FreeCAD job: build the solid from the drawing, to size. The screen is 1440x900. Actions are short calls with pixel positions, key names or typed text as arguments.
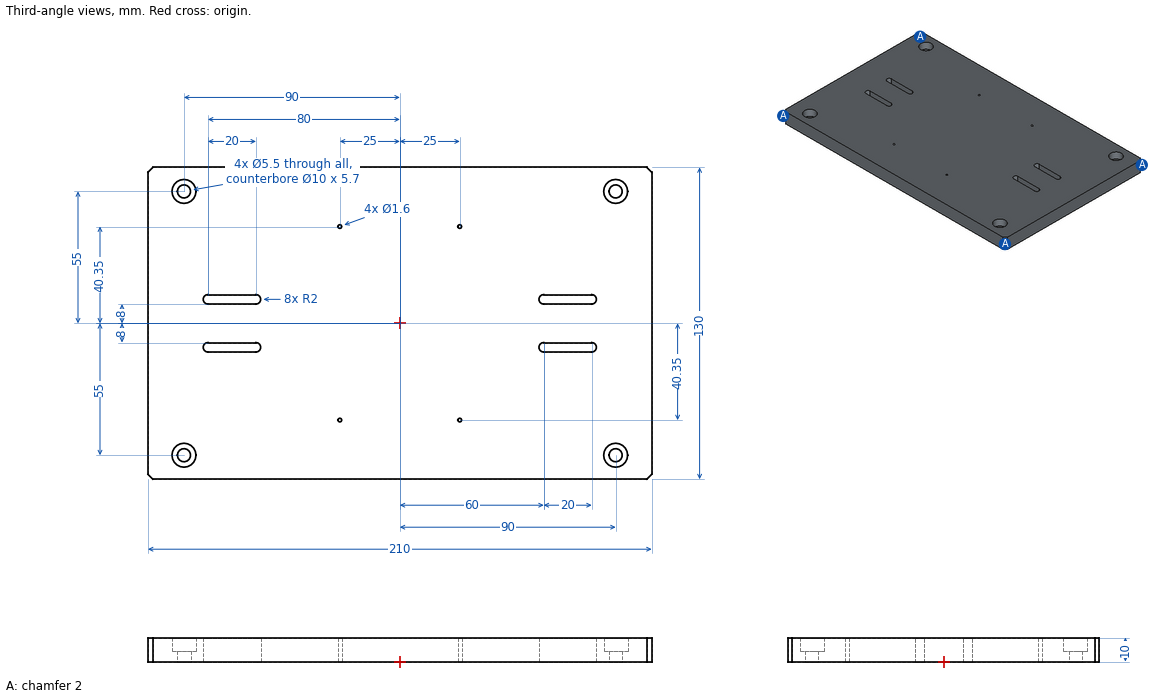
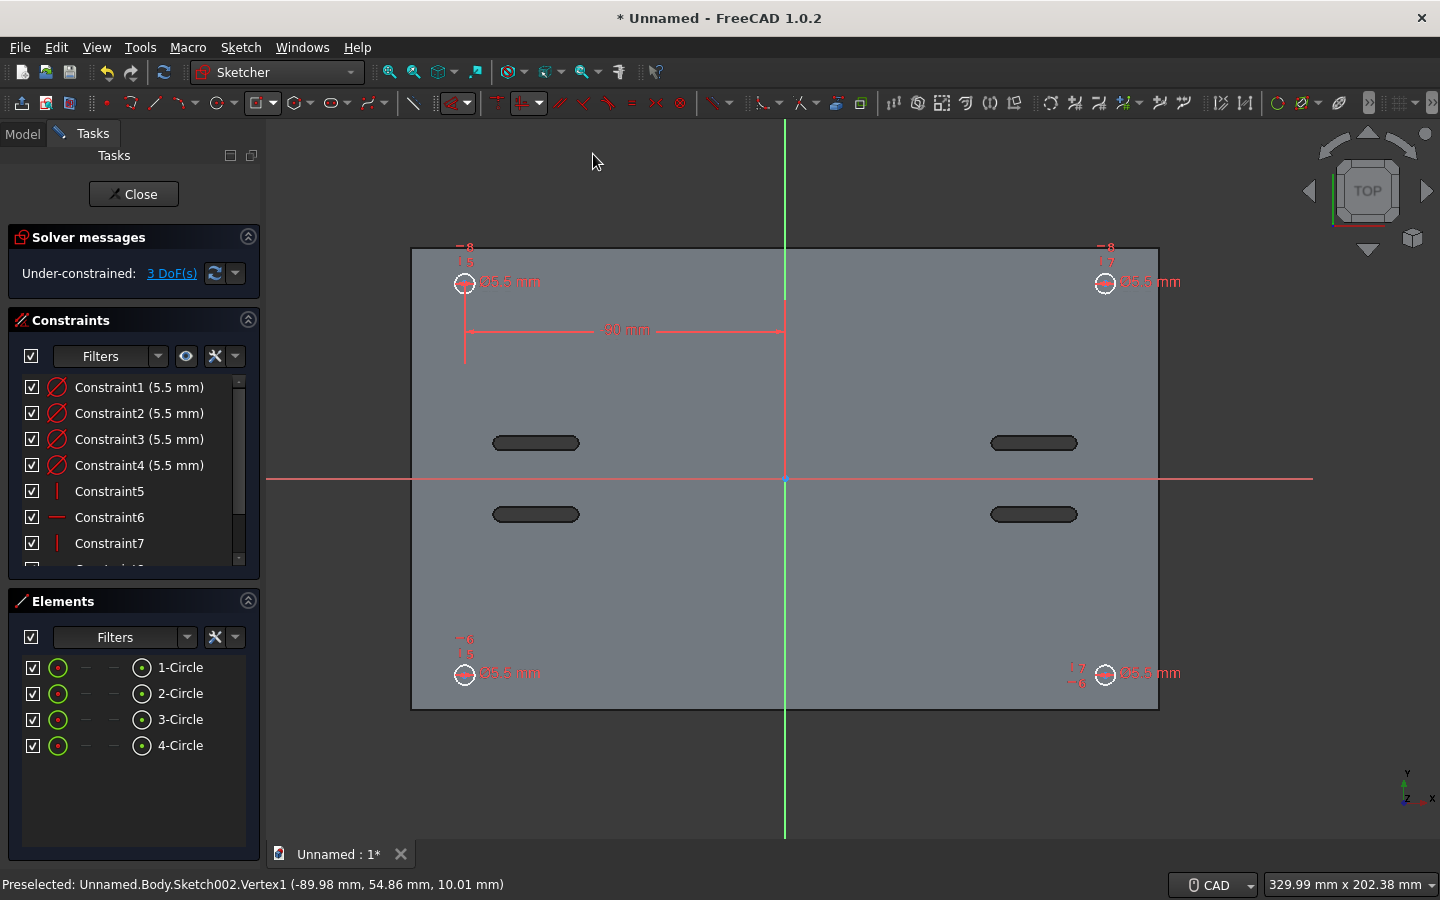
click(465, 284)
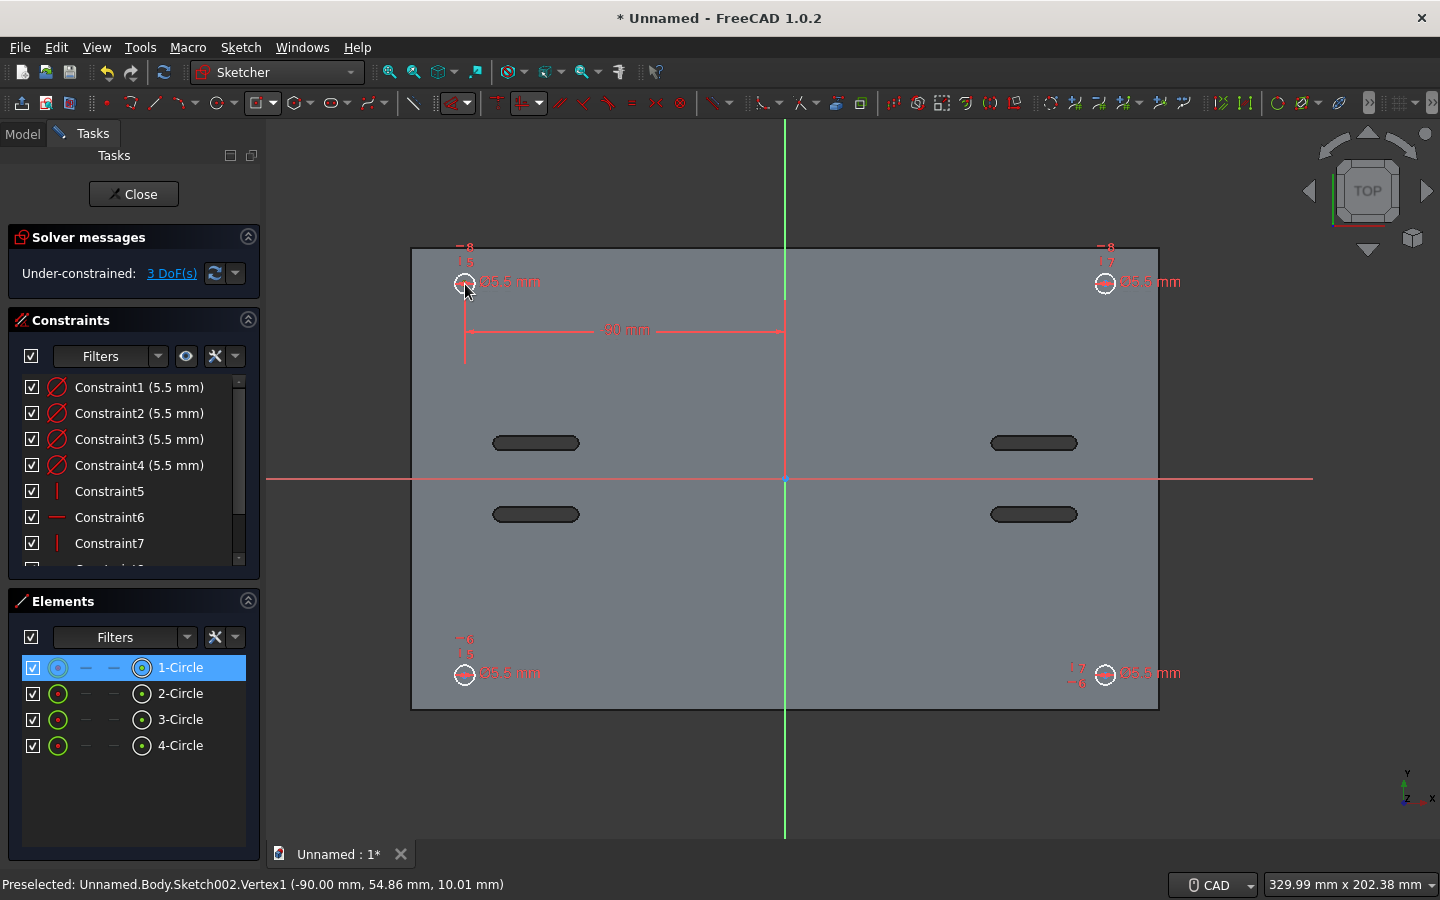
key(i)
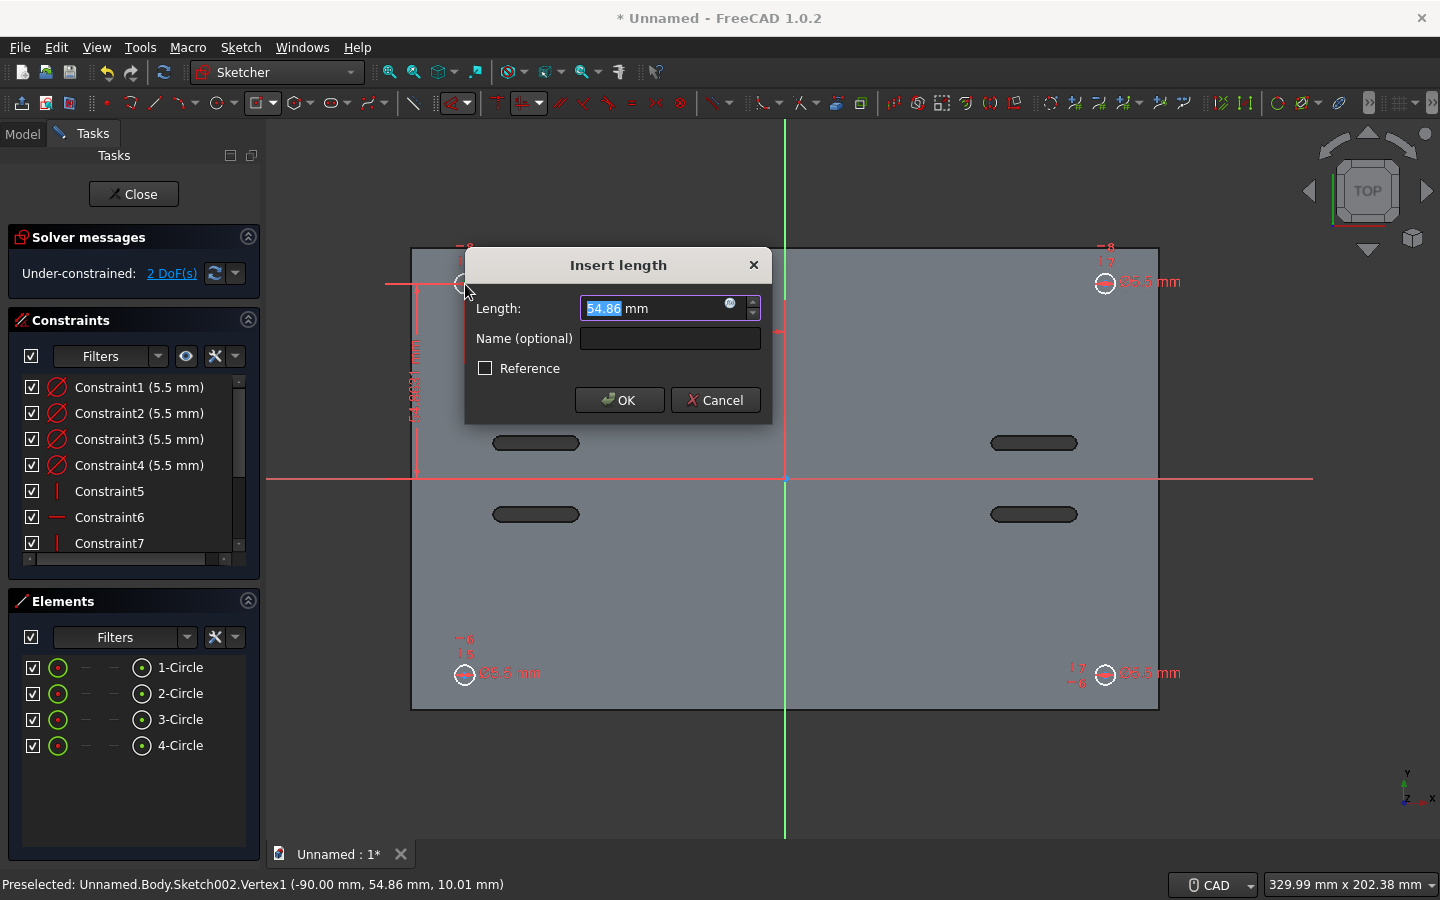
text(55)
key(Return)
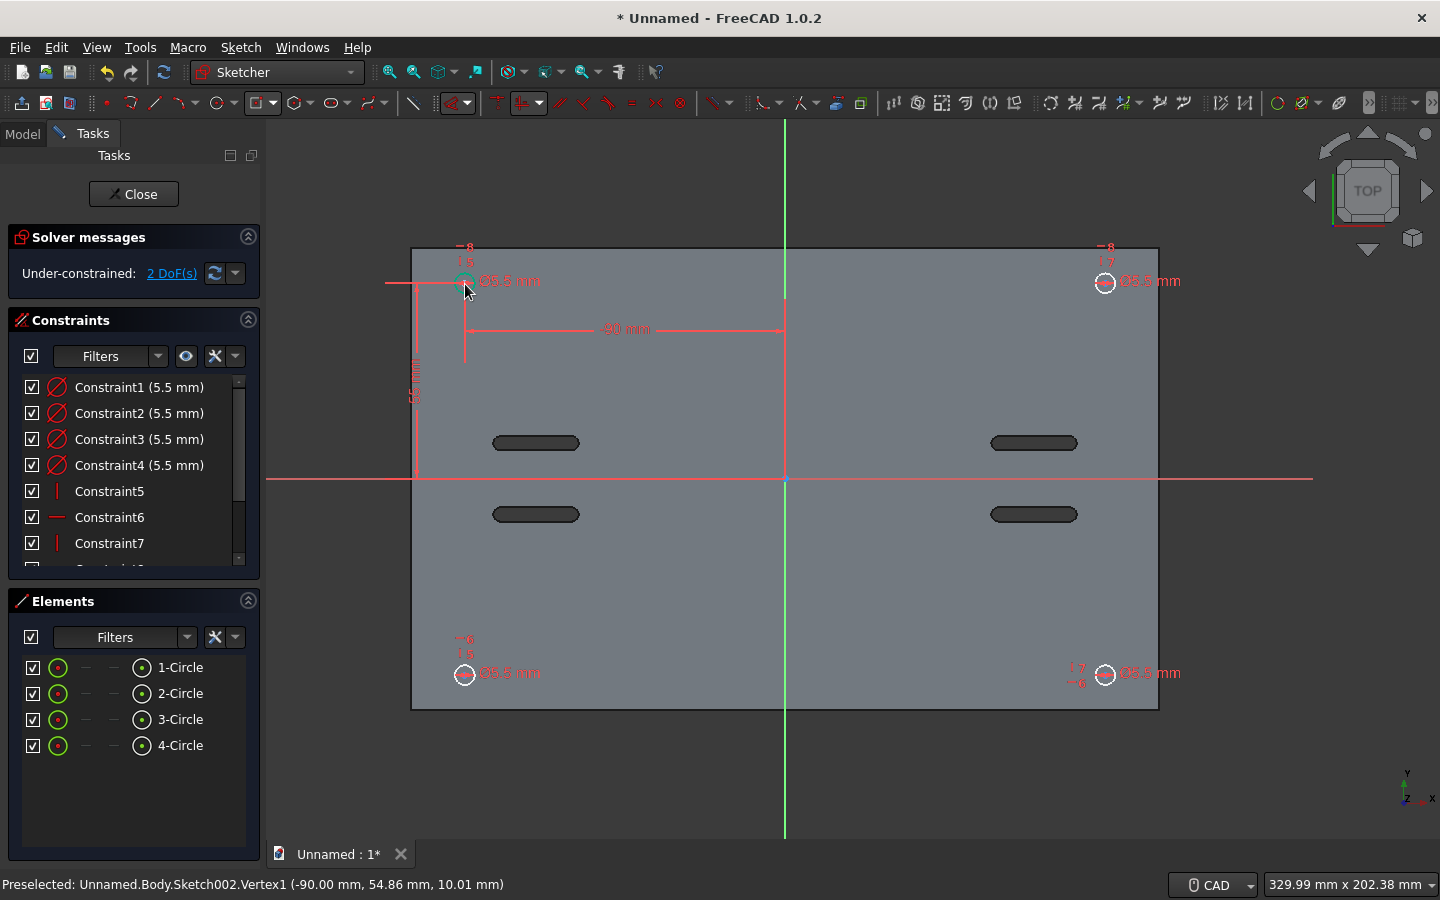
click(465, 675)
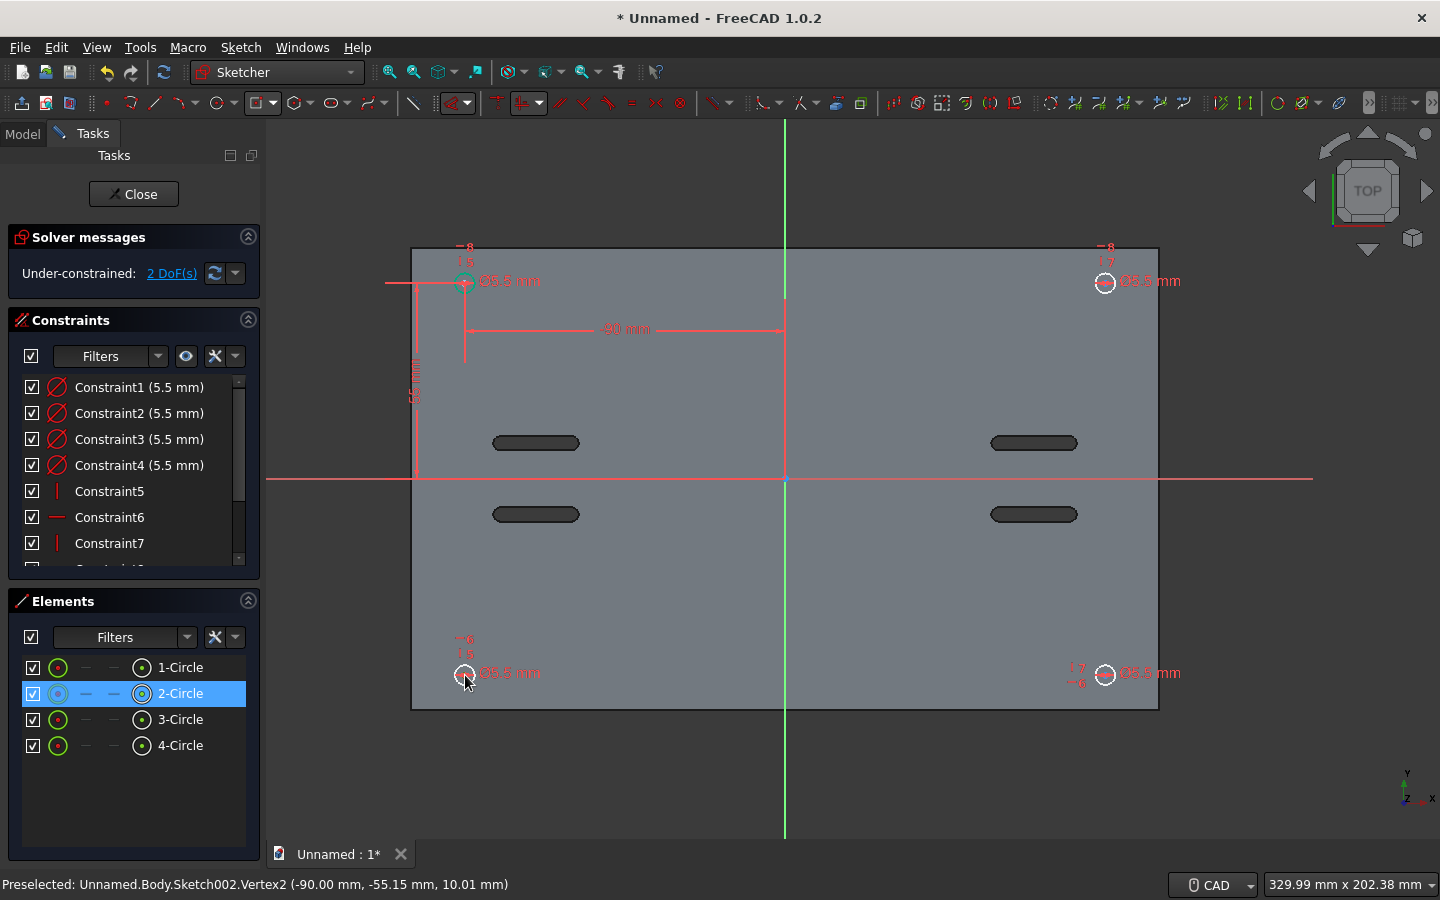
key(i)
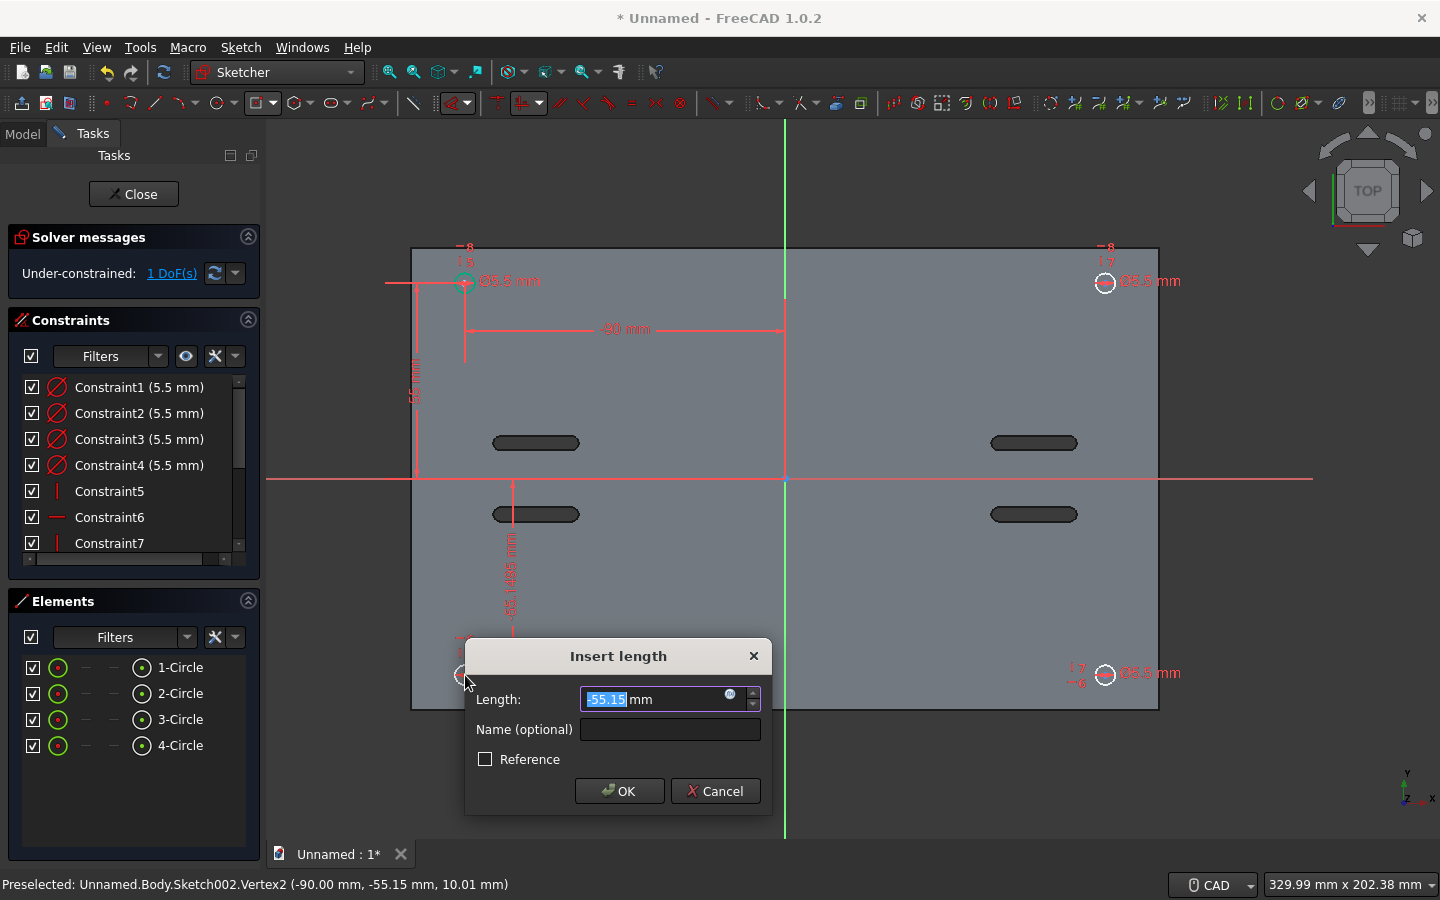
text(-55)
key(Return)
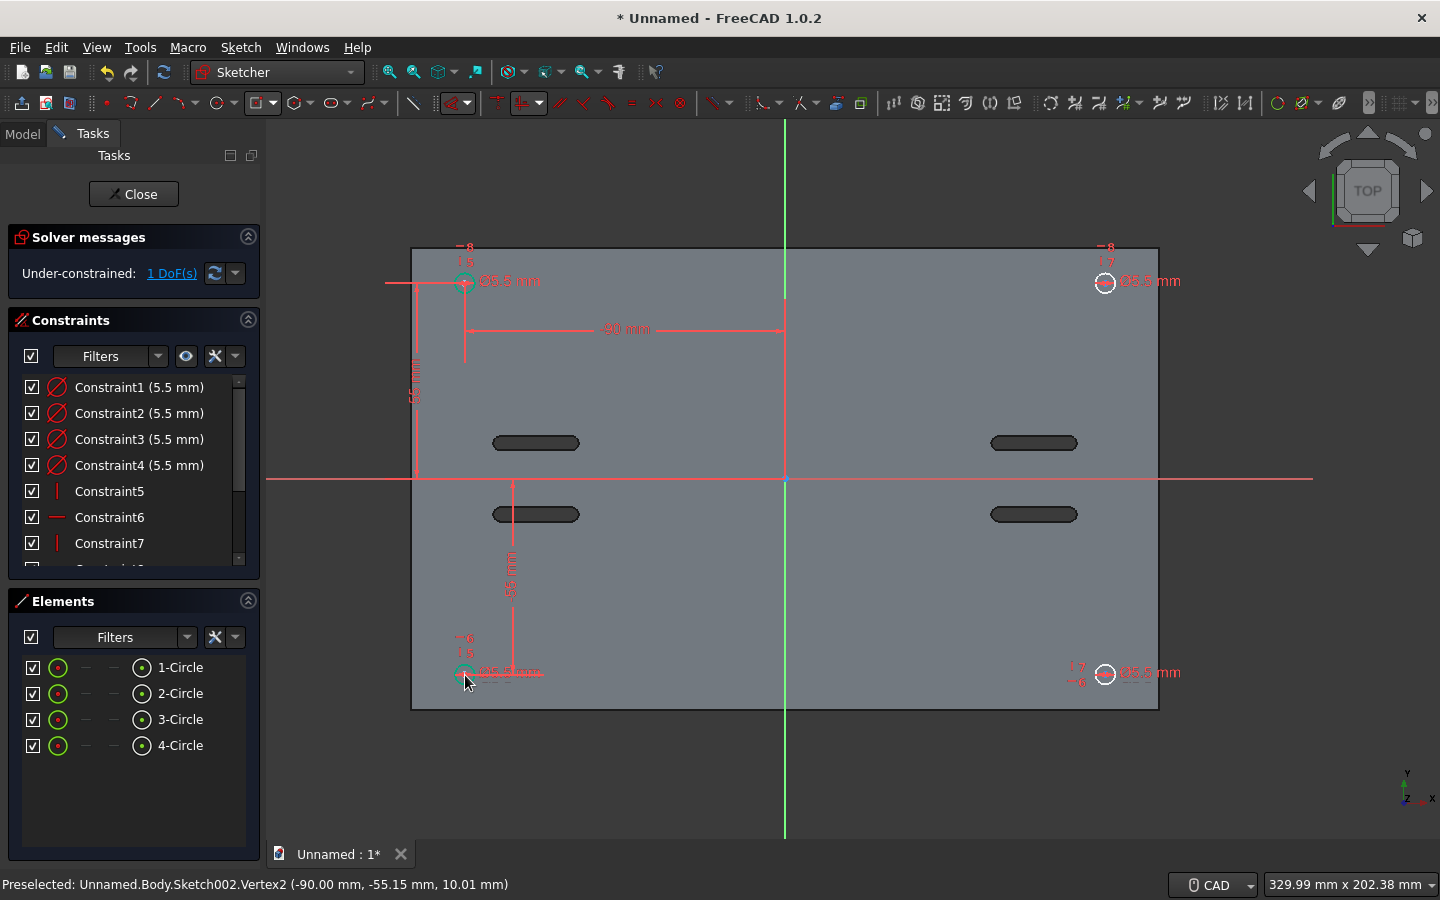
click(1105, 675)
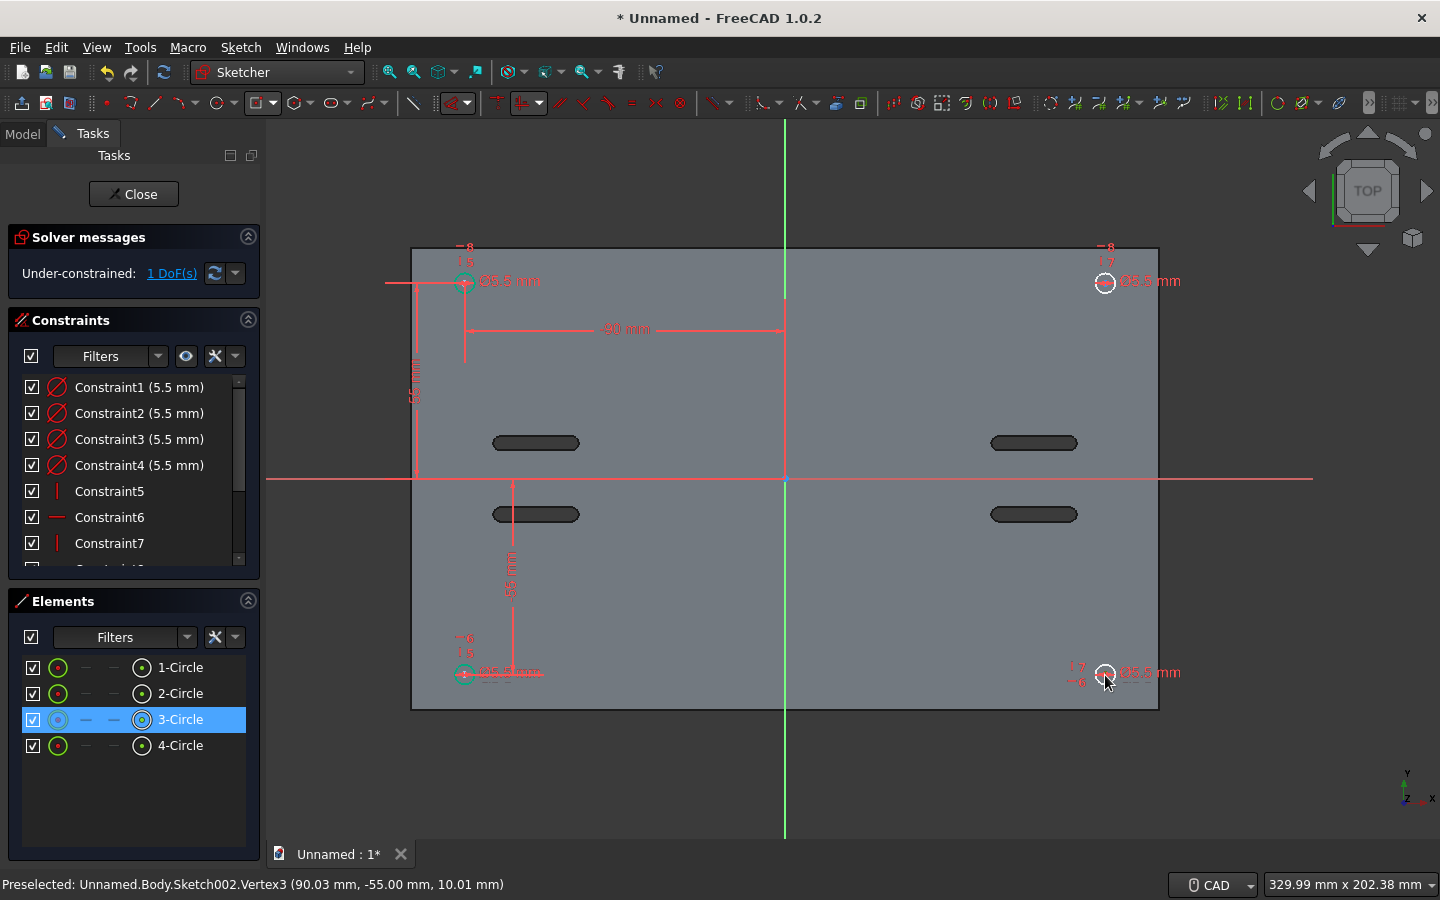
click(470, 104)